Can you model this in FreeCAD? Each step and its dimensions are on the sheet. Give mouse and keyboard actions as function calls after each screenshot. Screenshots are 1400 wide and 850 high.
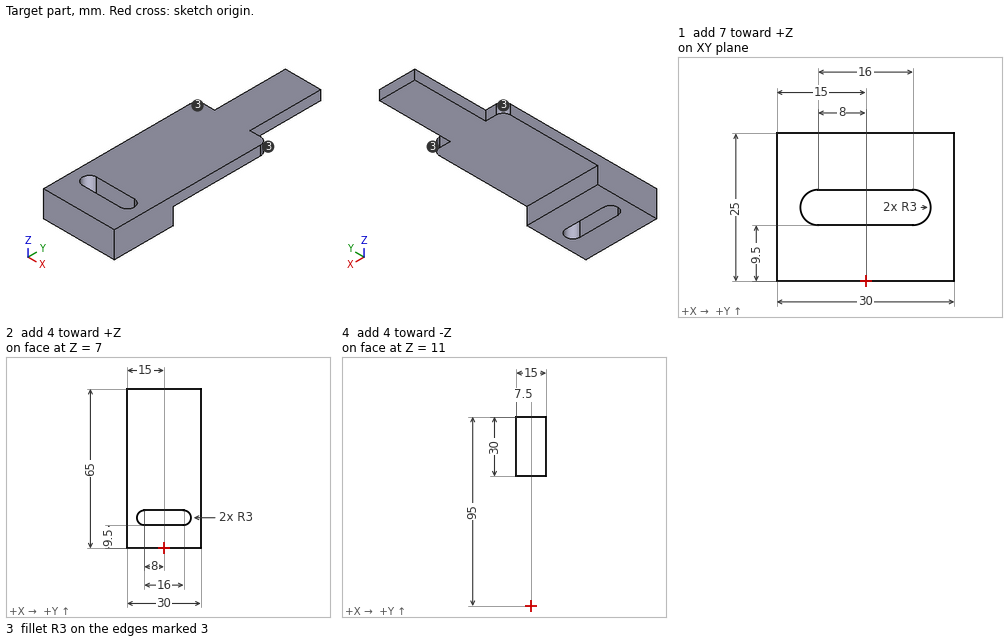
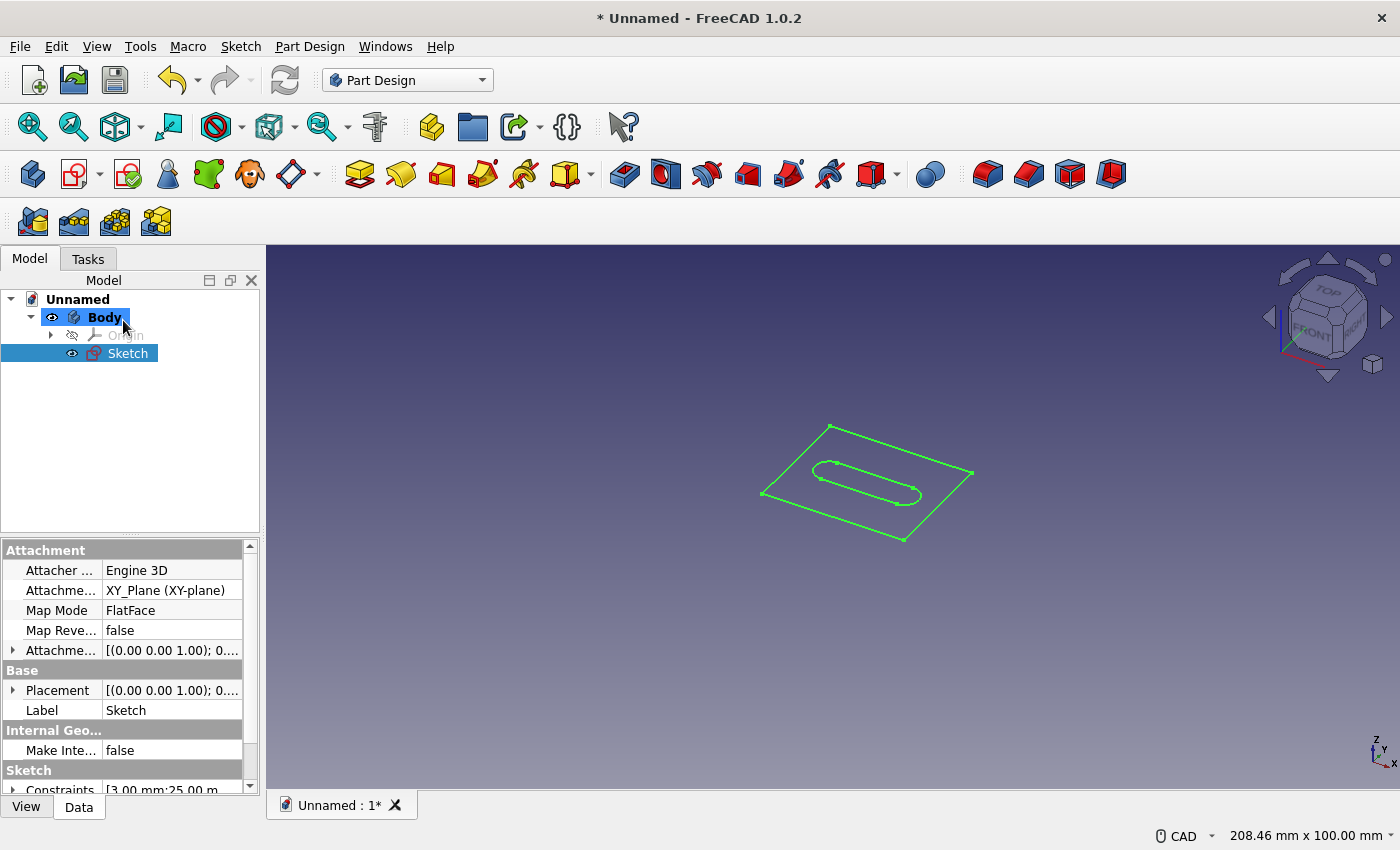
click(360, 174)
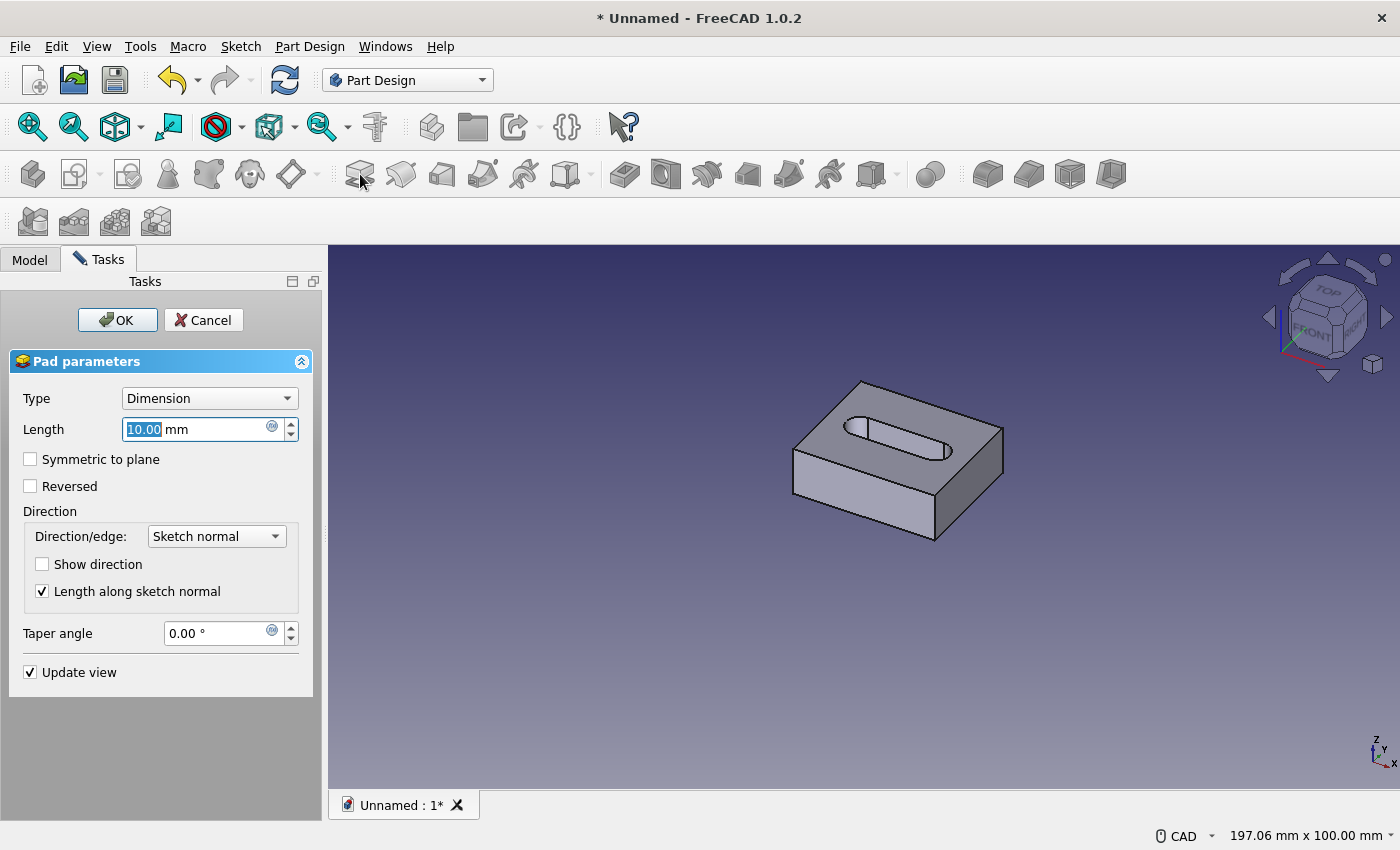
text(7)
key(Tab)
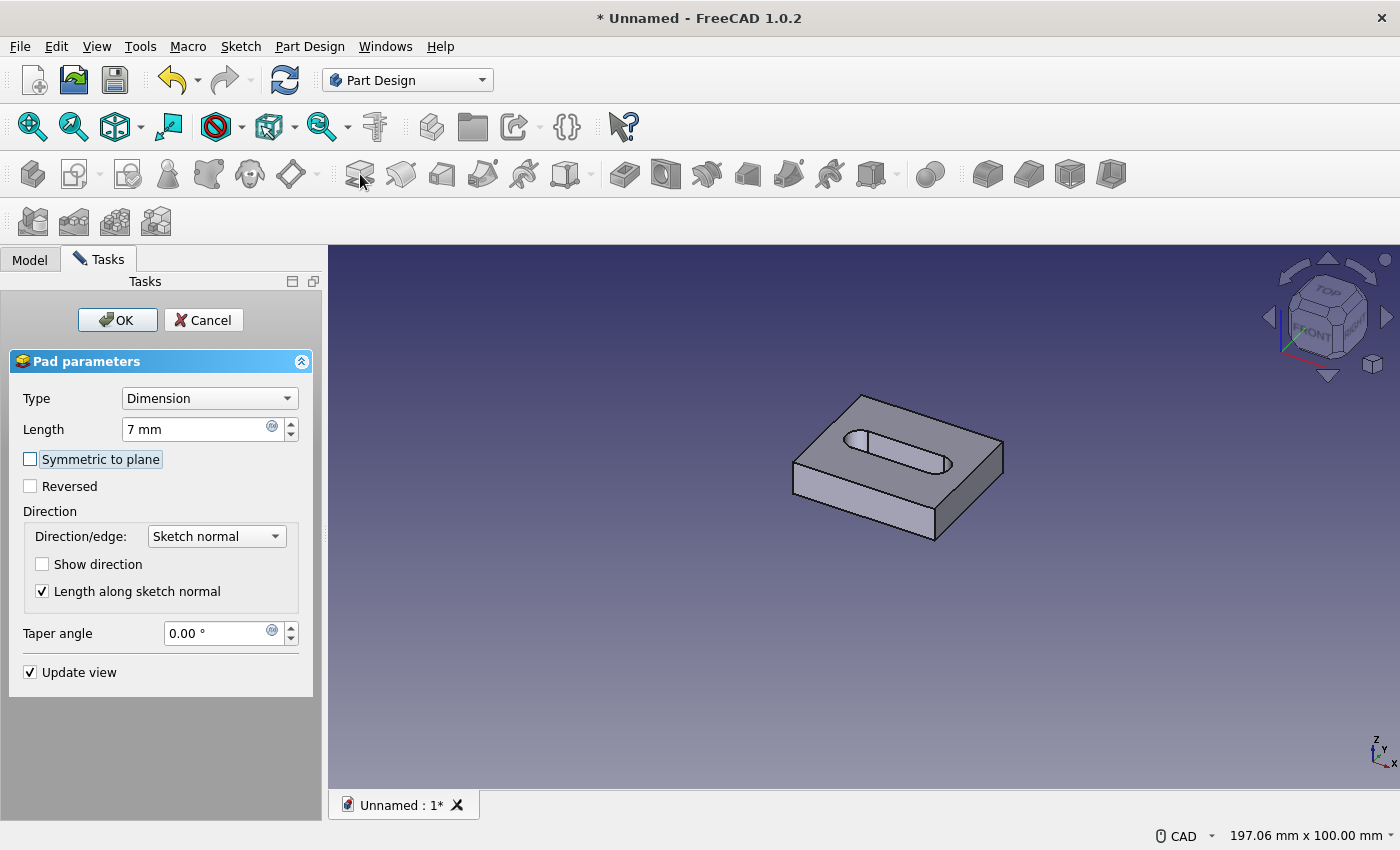
click(118, 320)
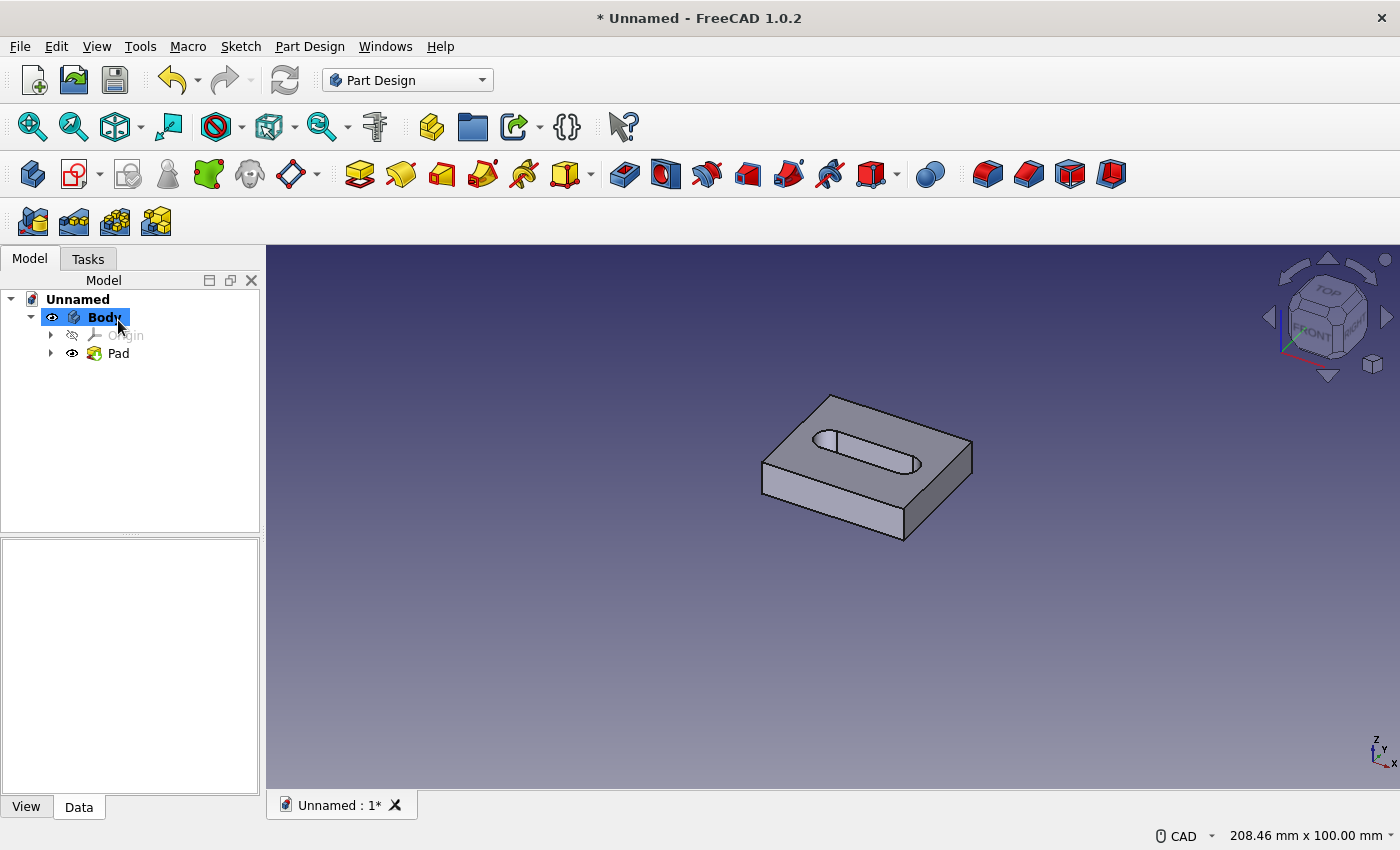
click(33, 128)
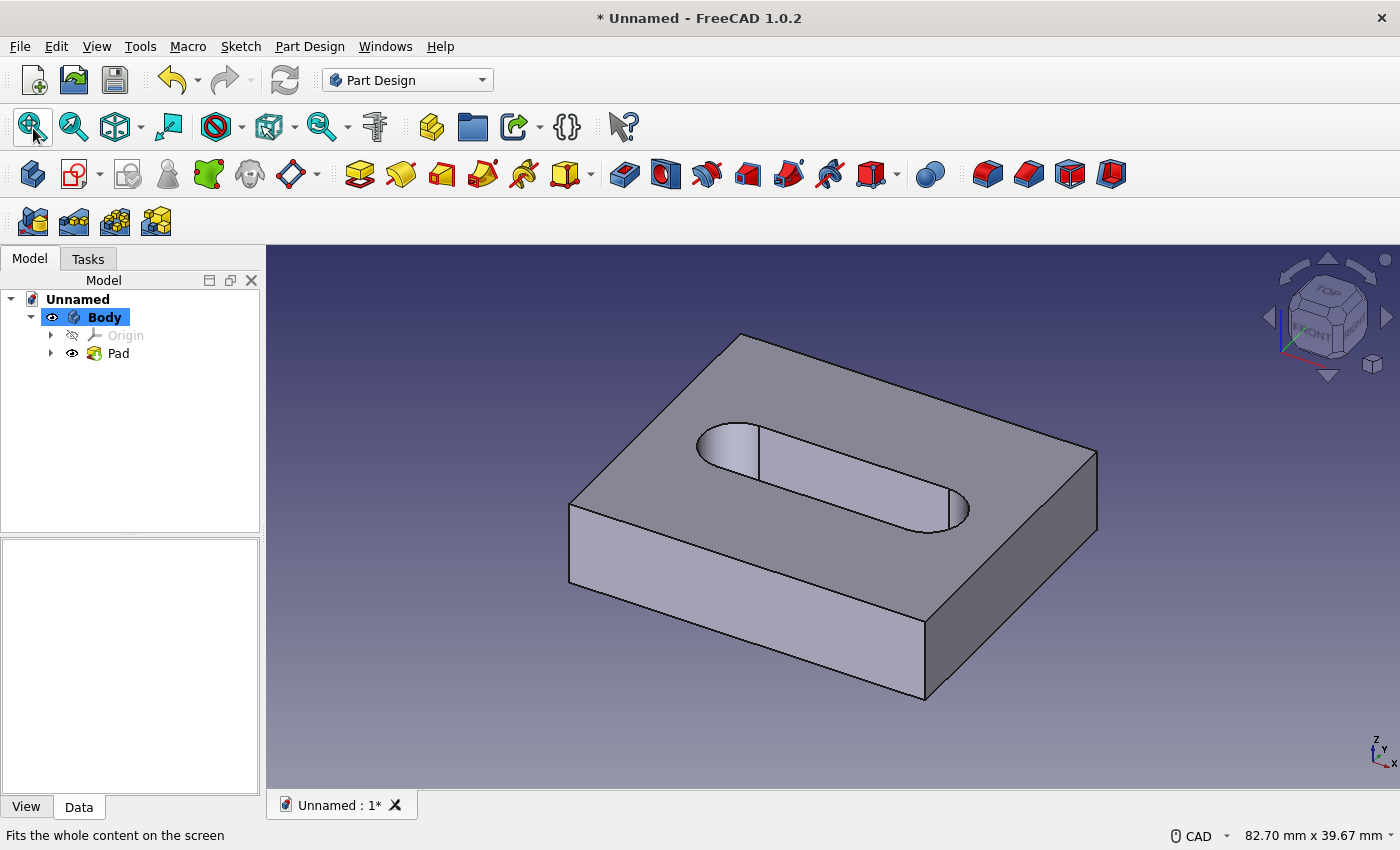
click(886, 559)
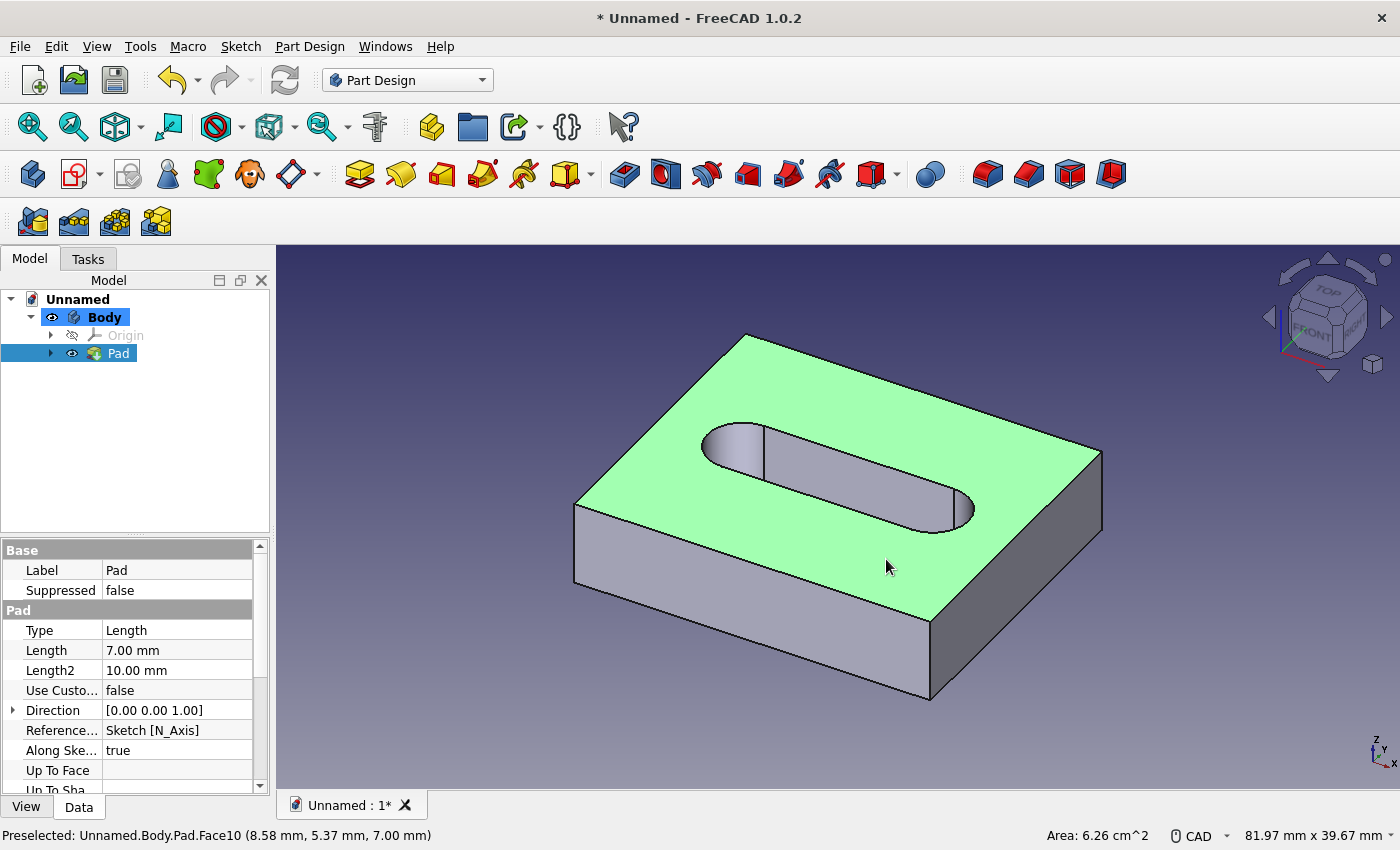
click(74, 174)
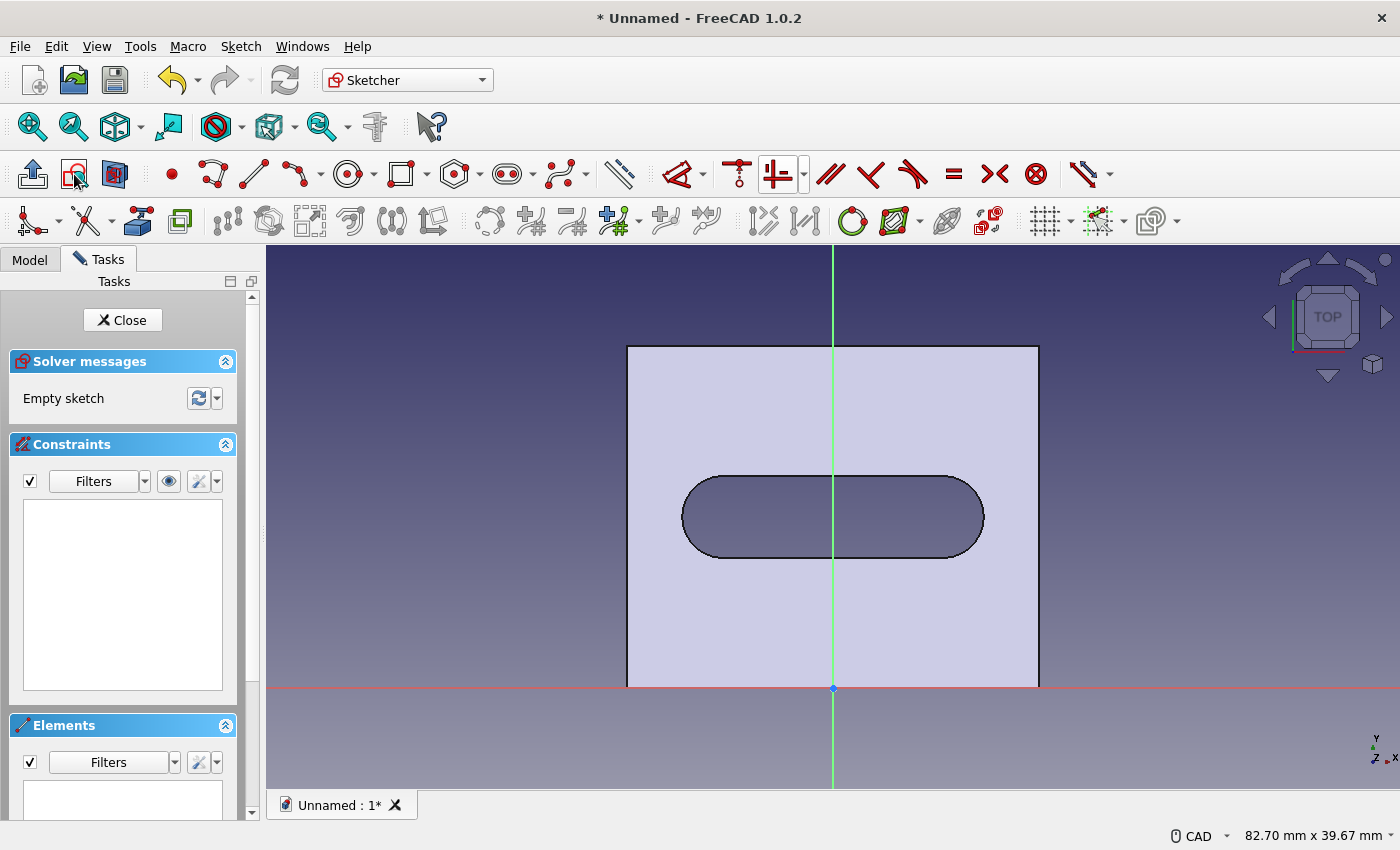
scroll(725, 677, down, 5)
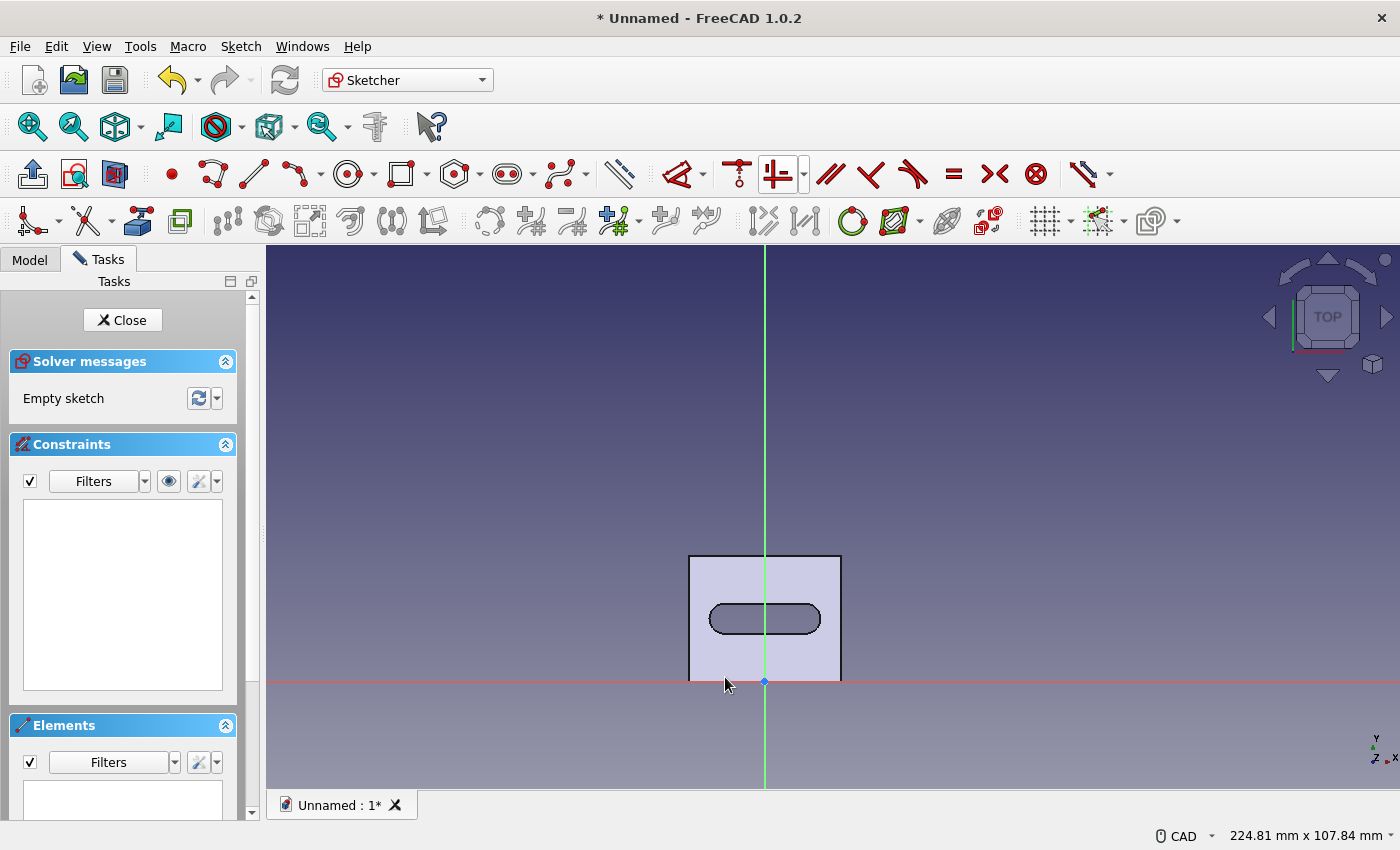
click(400, 174)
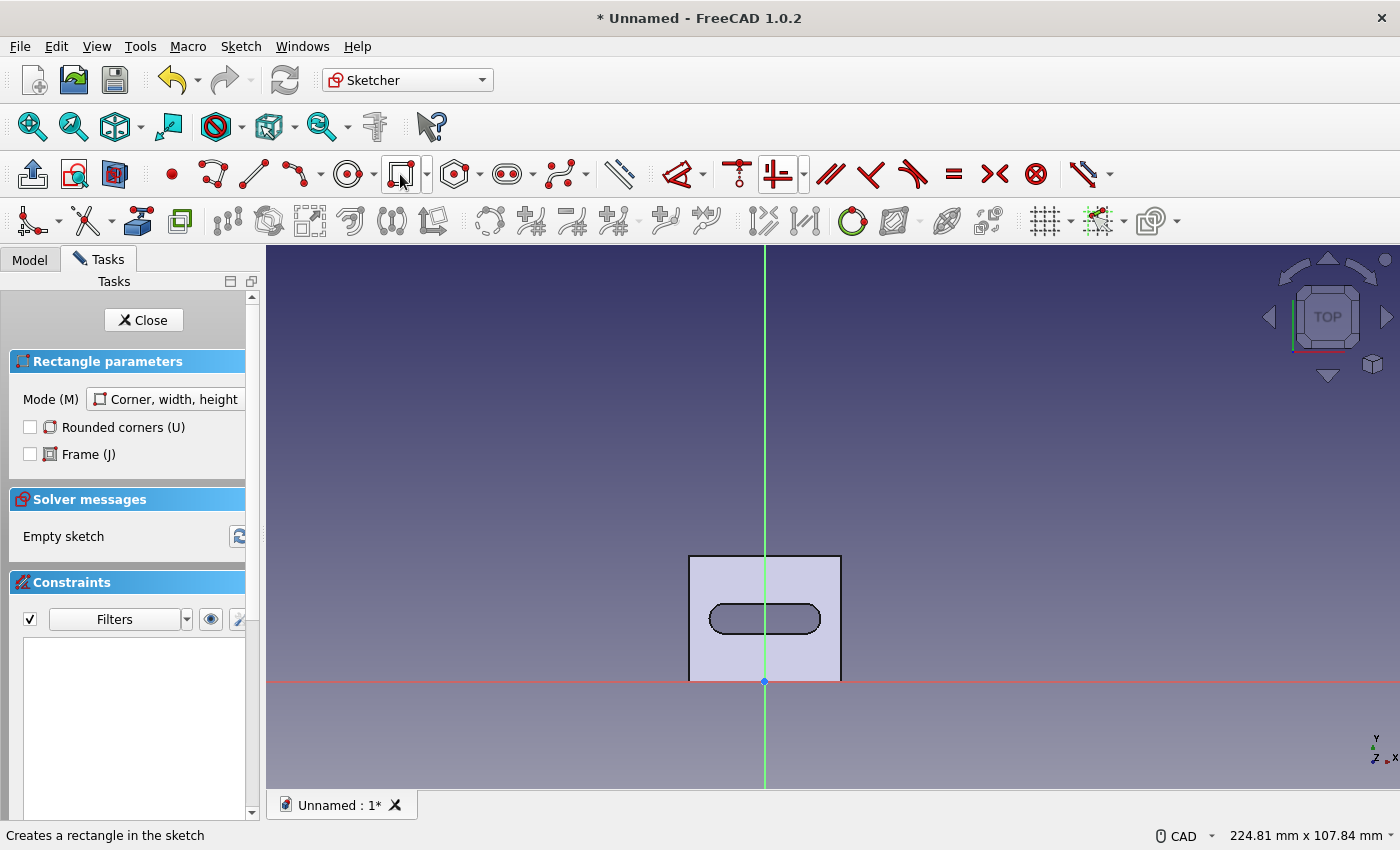
click(689, 354)
click(841, 682)